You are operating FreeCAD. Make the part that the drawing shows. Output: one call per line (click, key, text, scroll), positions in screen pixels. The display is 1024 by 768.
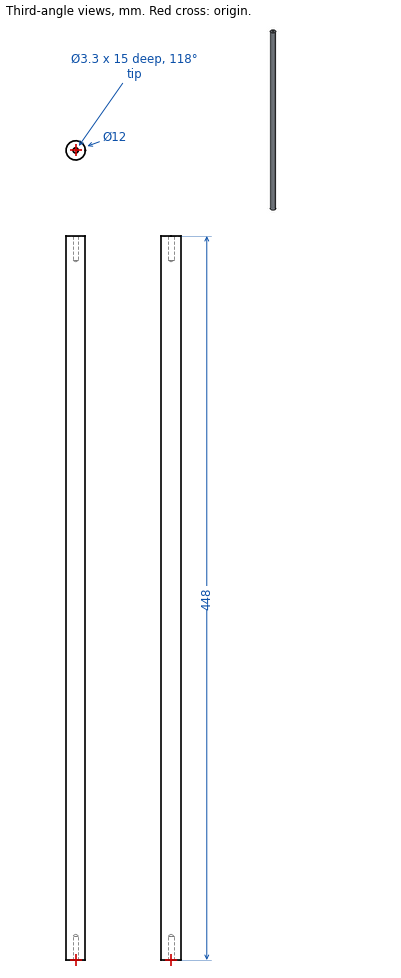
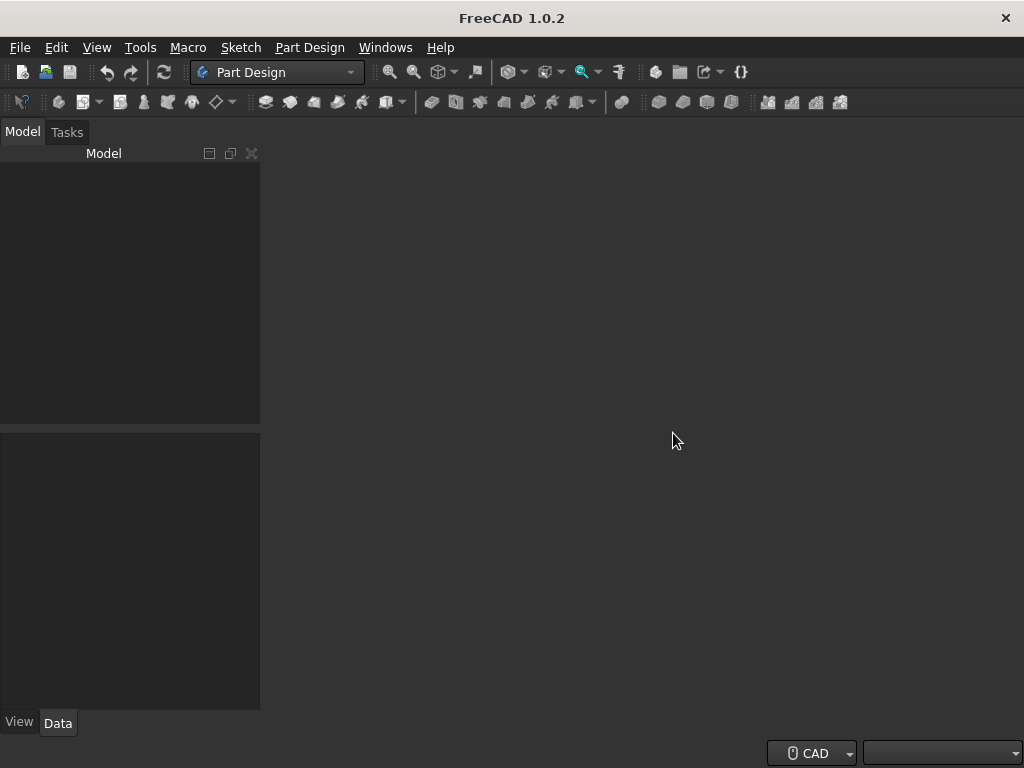
click(22, 72)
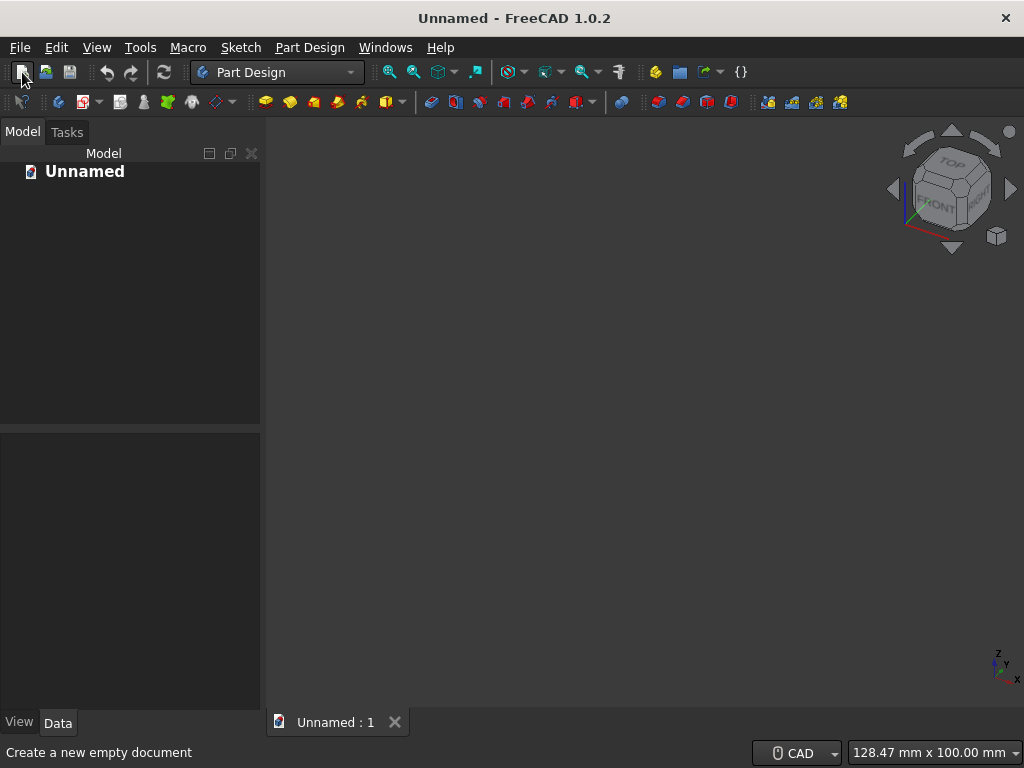
click(84, 102)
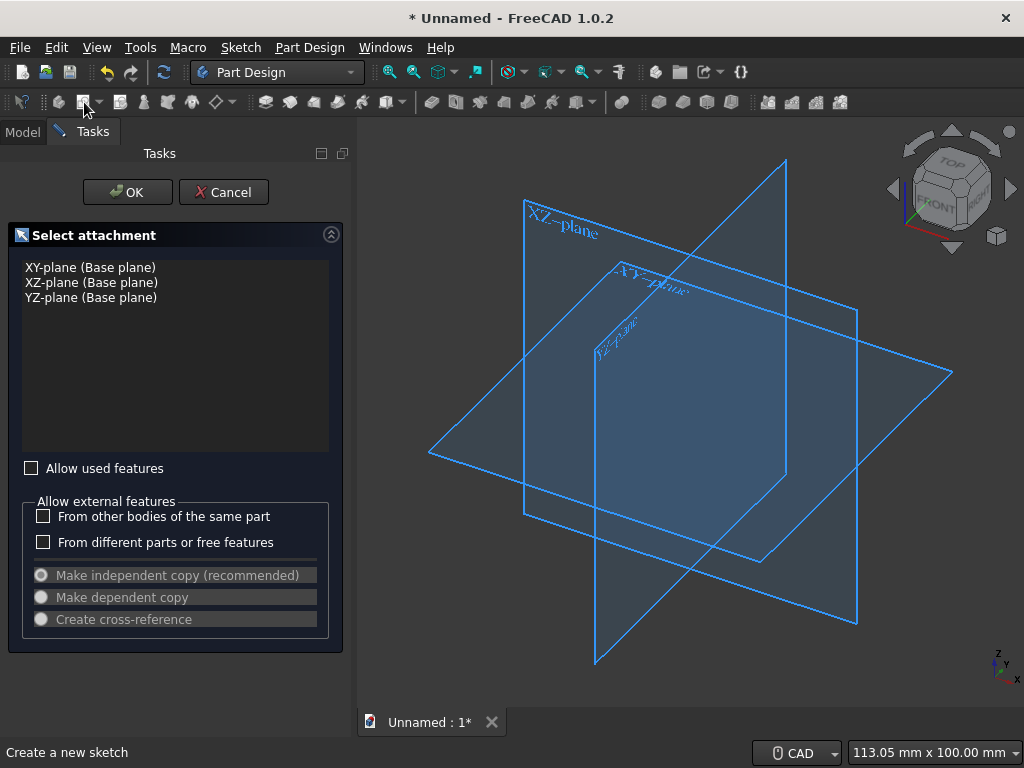
click(82, 268)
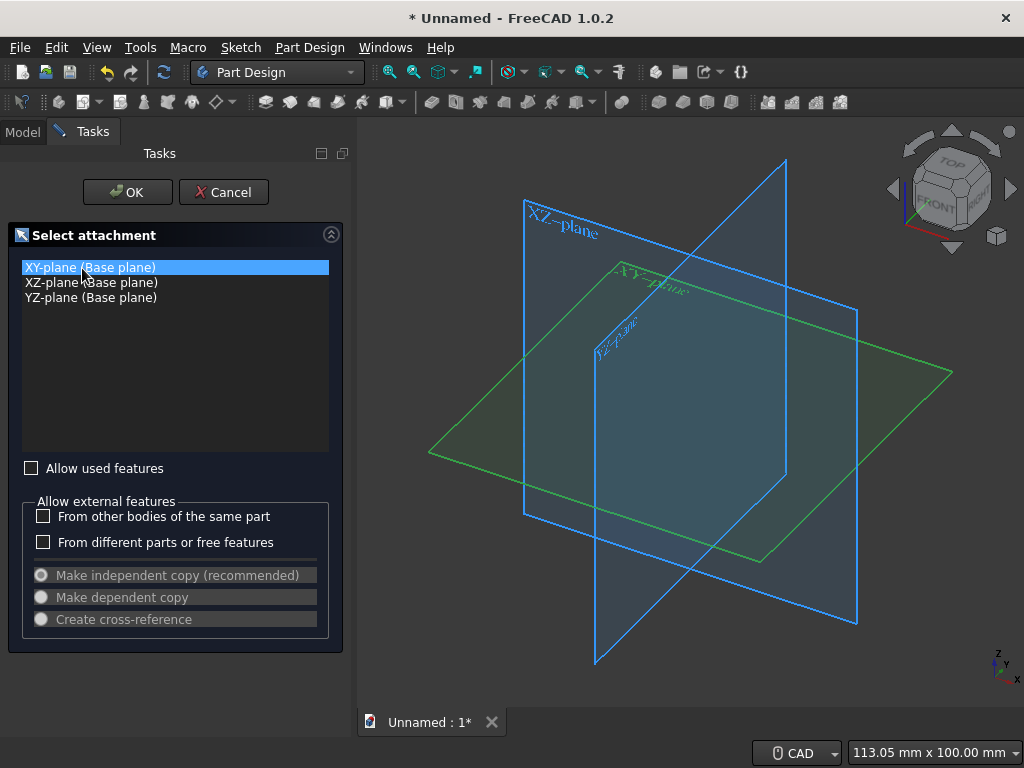
click(128, 192)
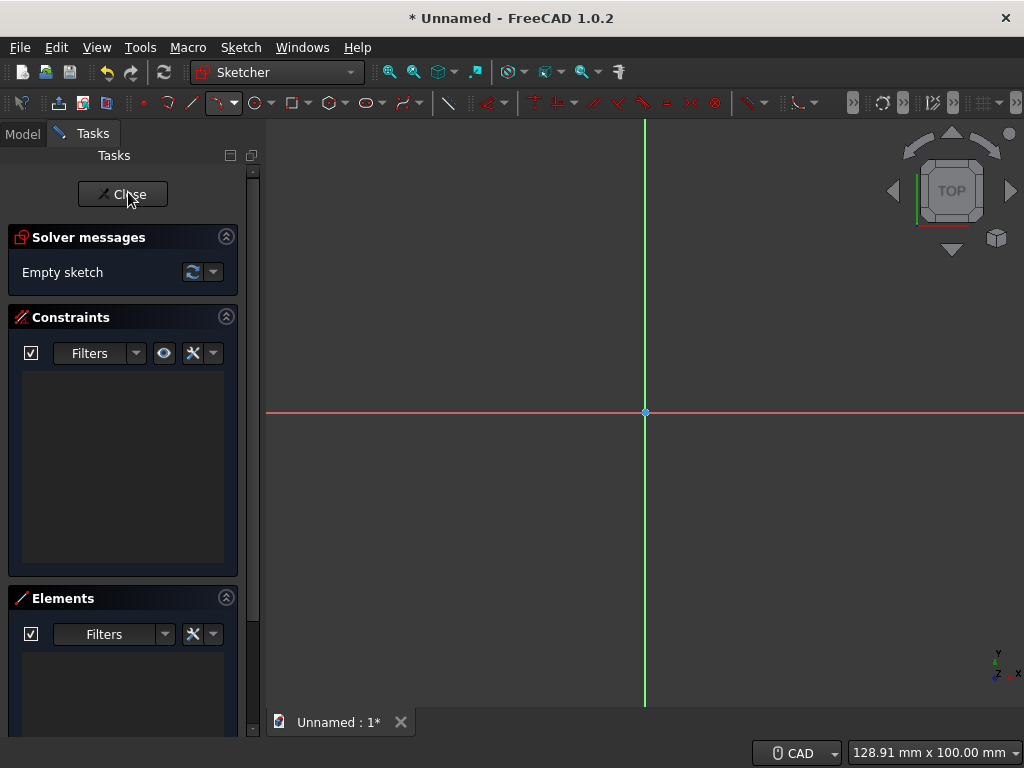
scroll(662, 413, up, 8)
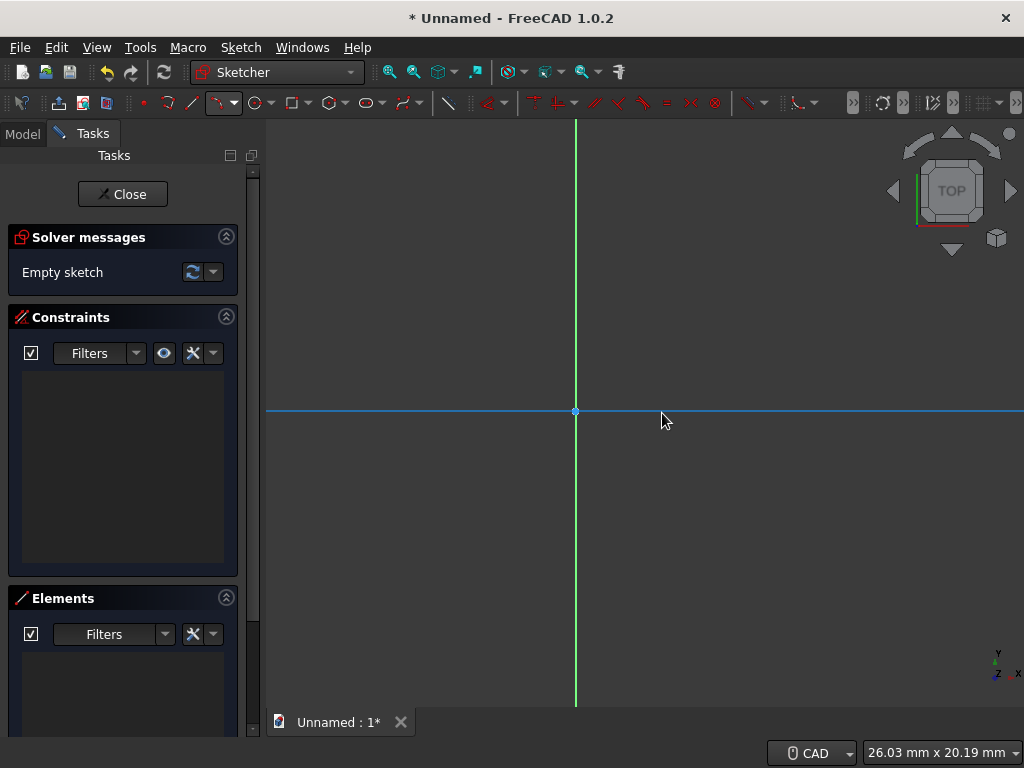
click(256, 104)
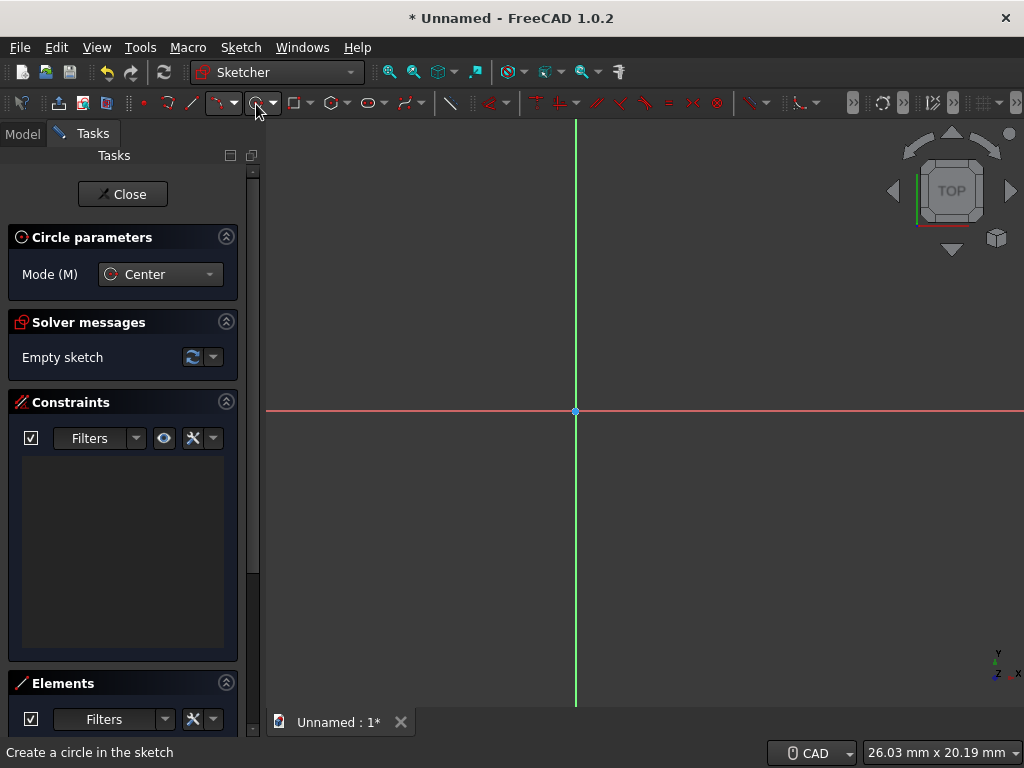
click(576, 411)
move(699, 287)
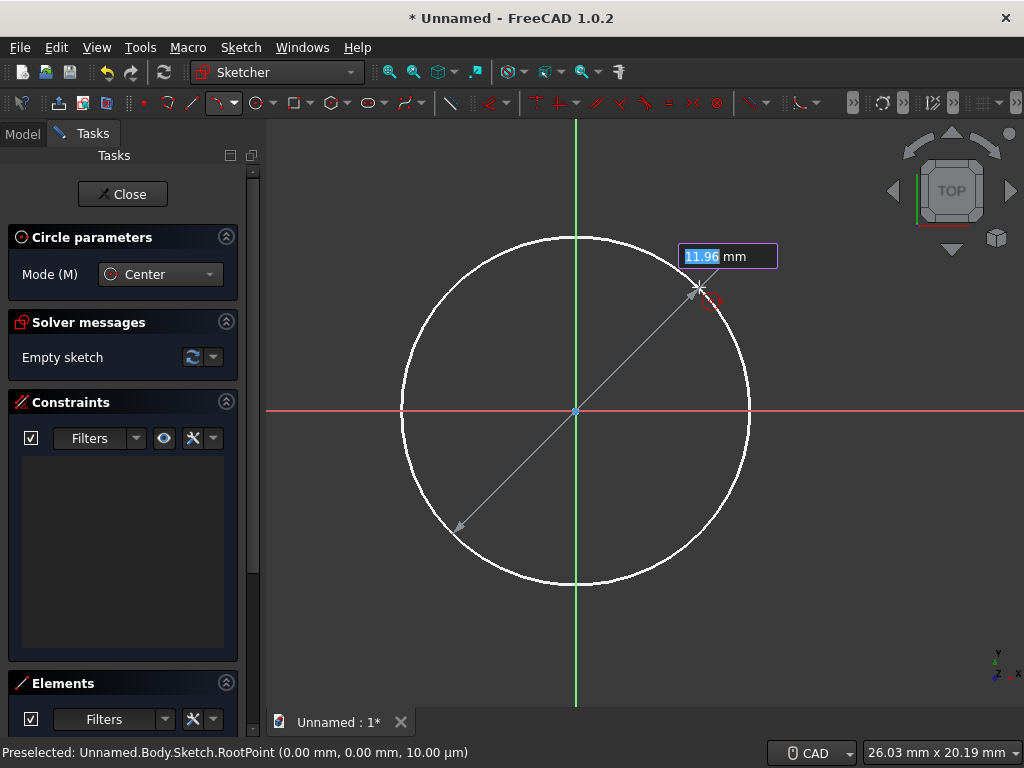
text(12)
key(Return)
key(Escape)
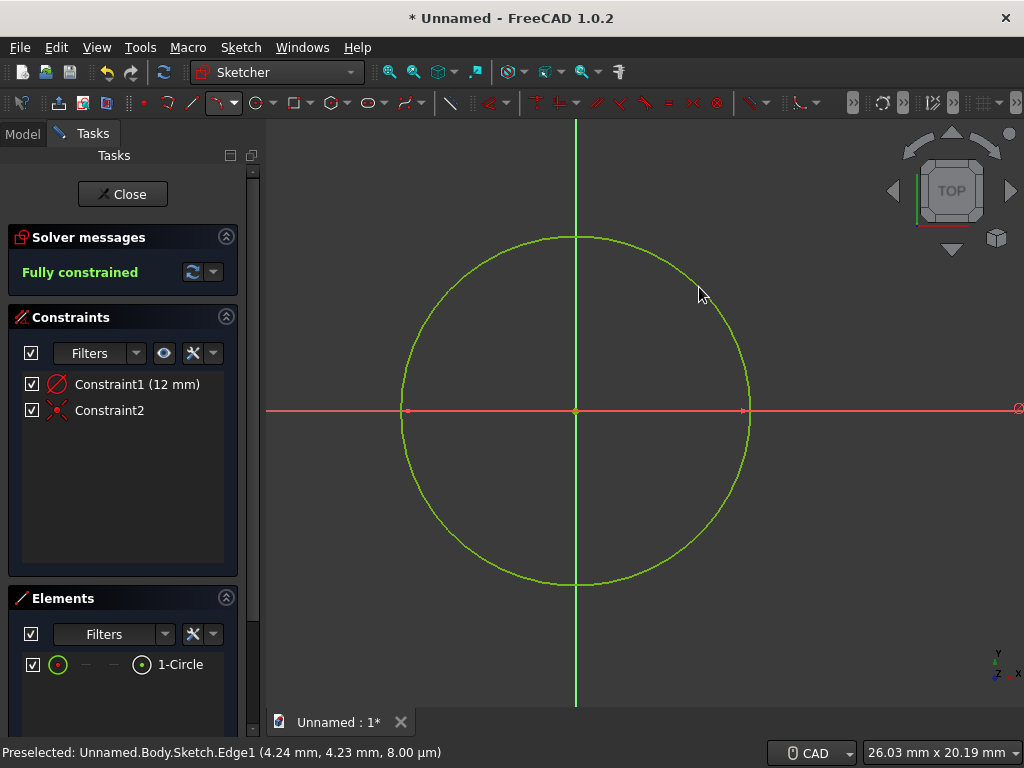
click(123, 194)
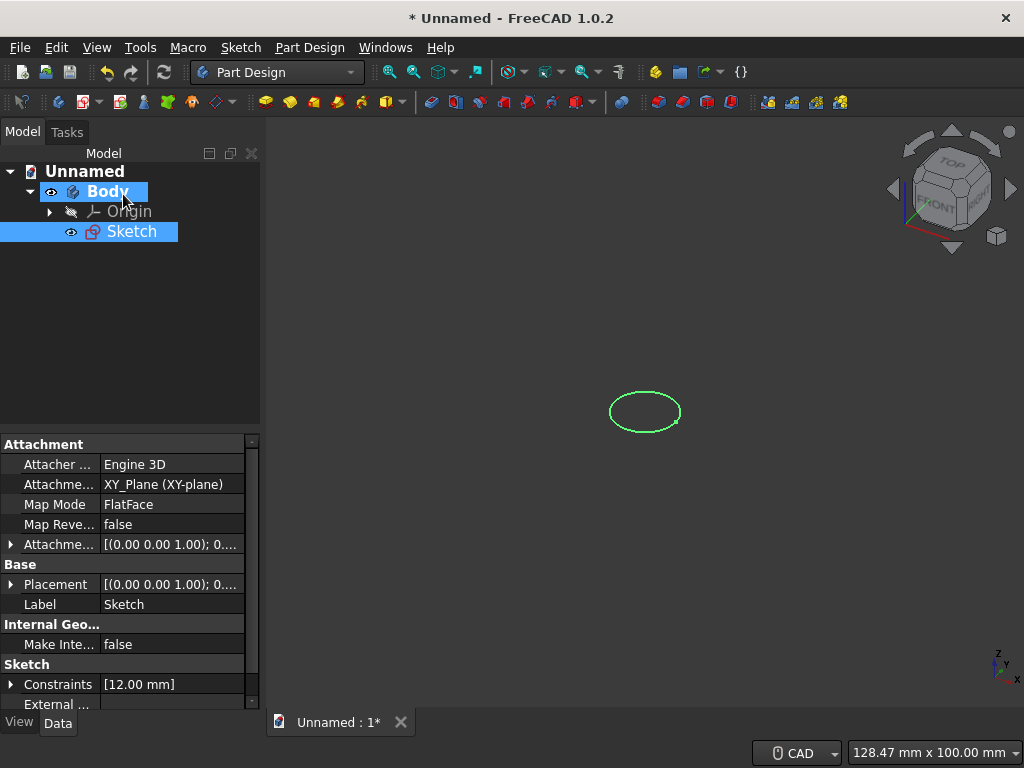
click(266, 102)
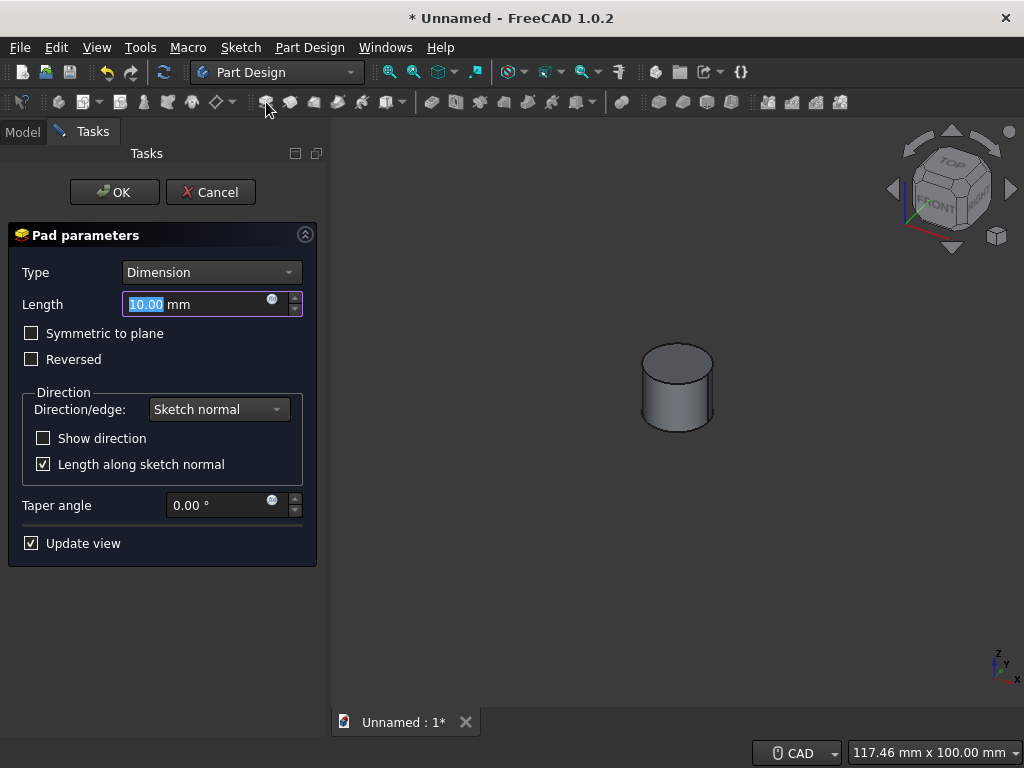
text(448)
key(Tab)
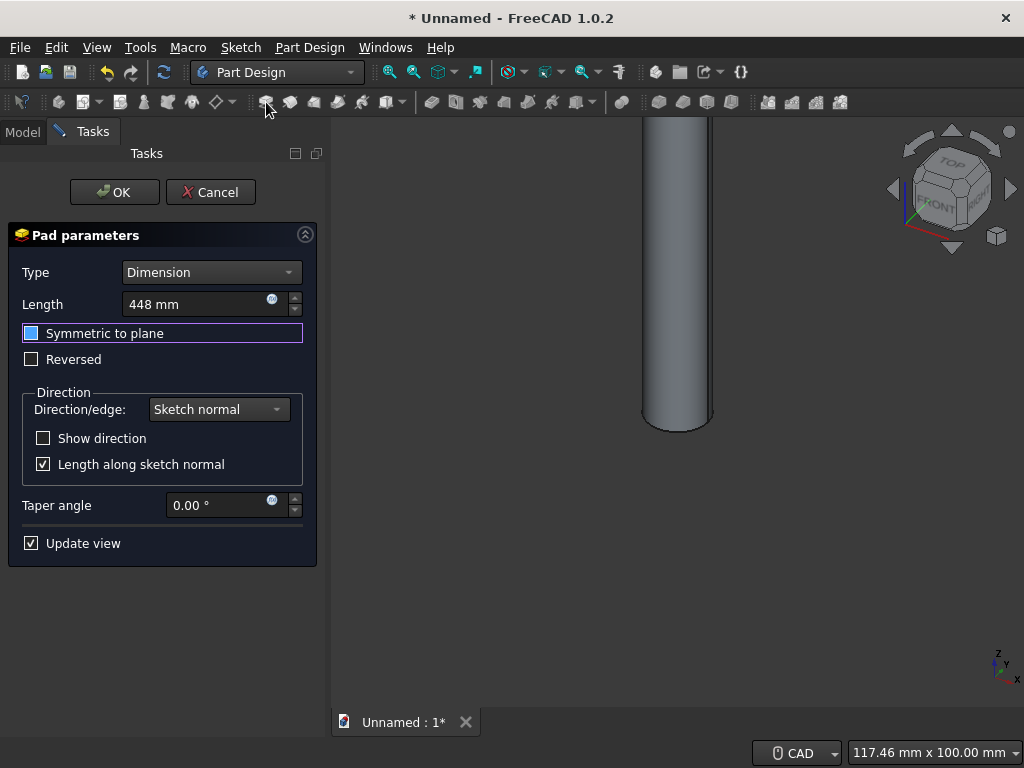
click(115, 192)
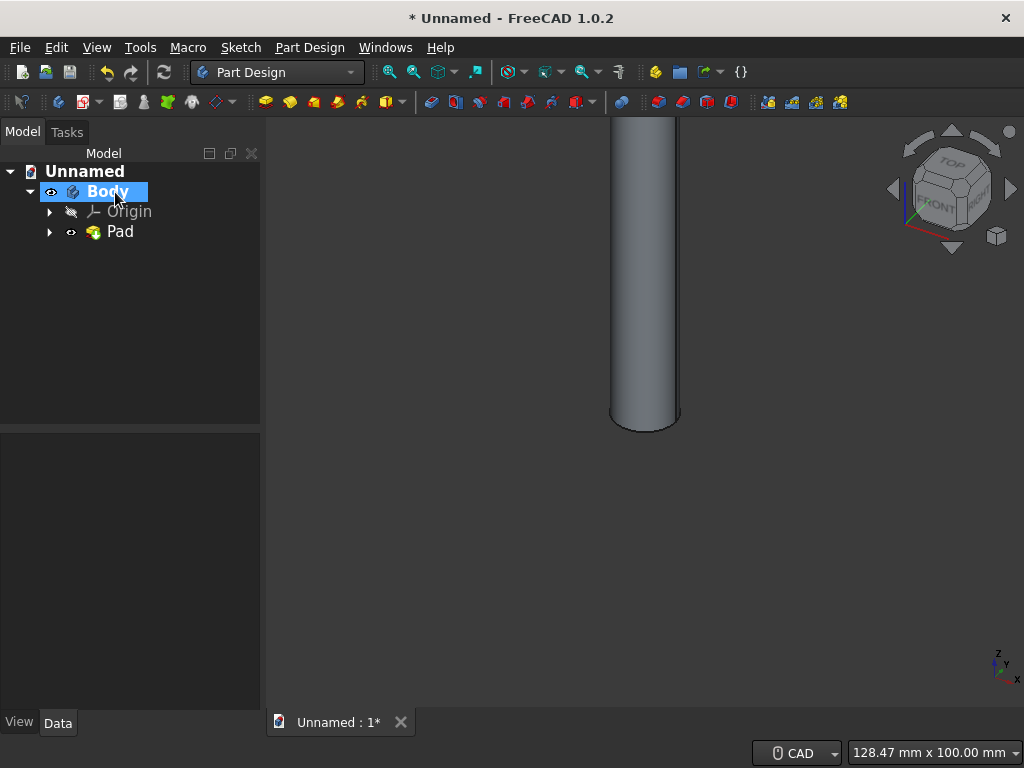
click(390, 72)